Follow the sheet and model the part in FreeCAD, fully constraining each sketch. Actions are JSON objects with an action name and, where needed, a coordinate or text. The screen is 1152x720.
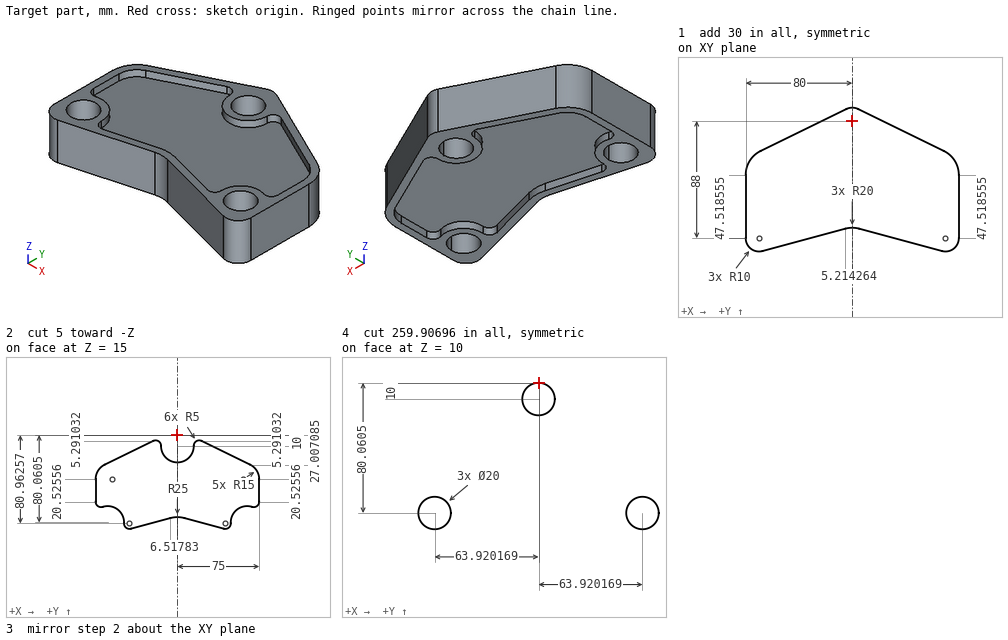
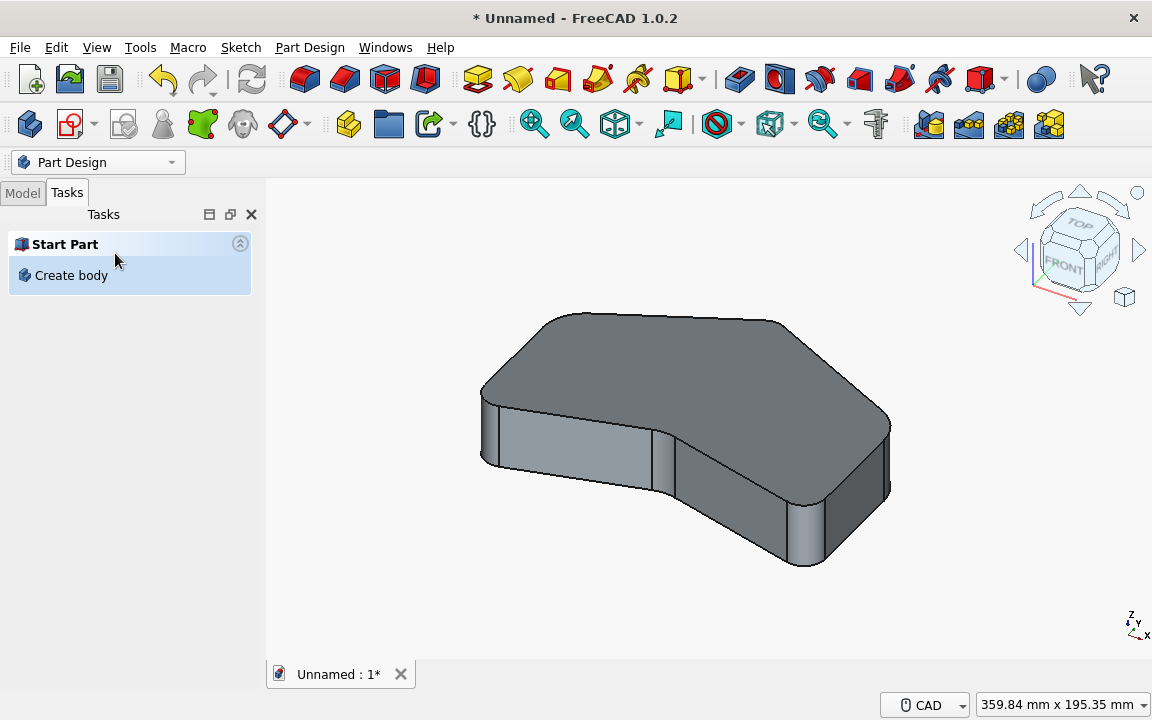
{"action": "left_click", "coordinate": [660, 371]}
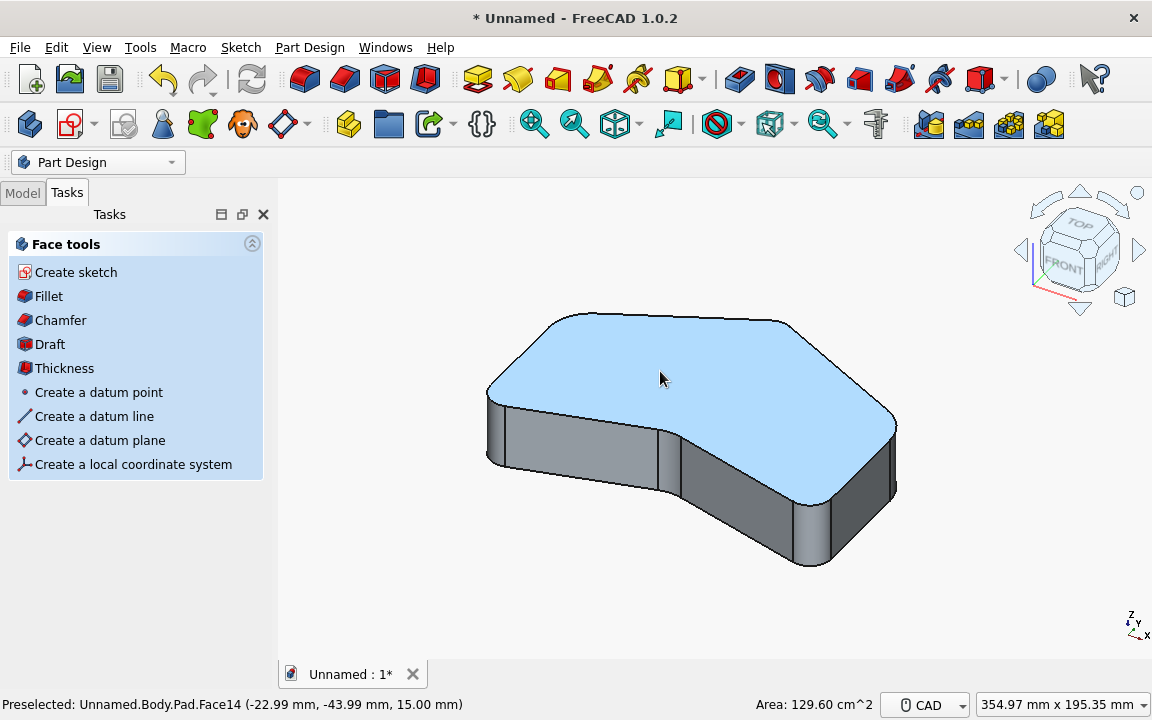
{"action": "left_click", "coordinate": [70, 124]}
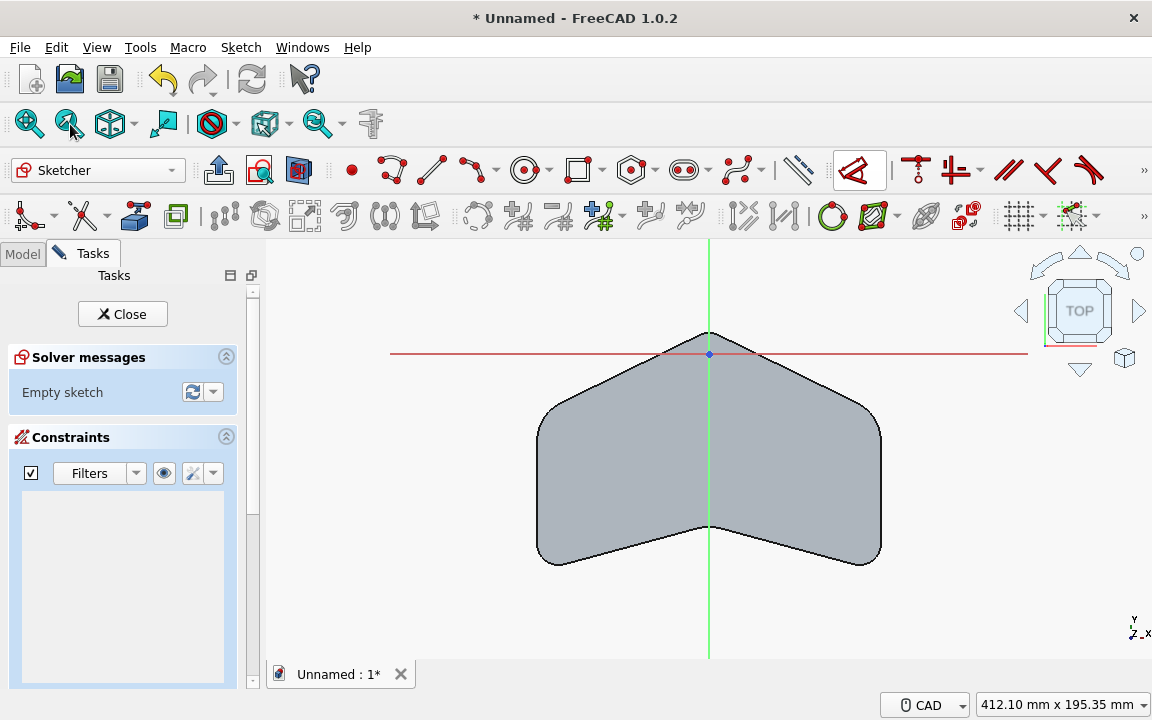
{"action": "scroll", "coordinate": [848, 442], "scroll_direction": "up", "scroll_amount": 2}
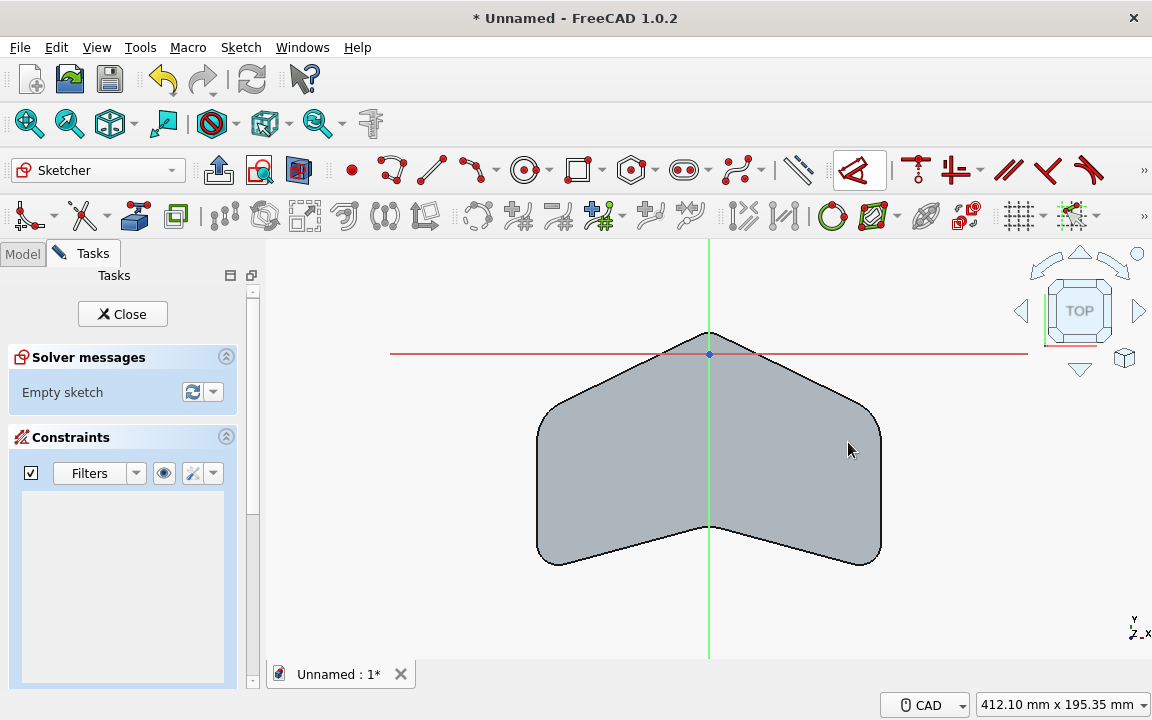
{"action": "left_click", "coordinate": [432, 170]}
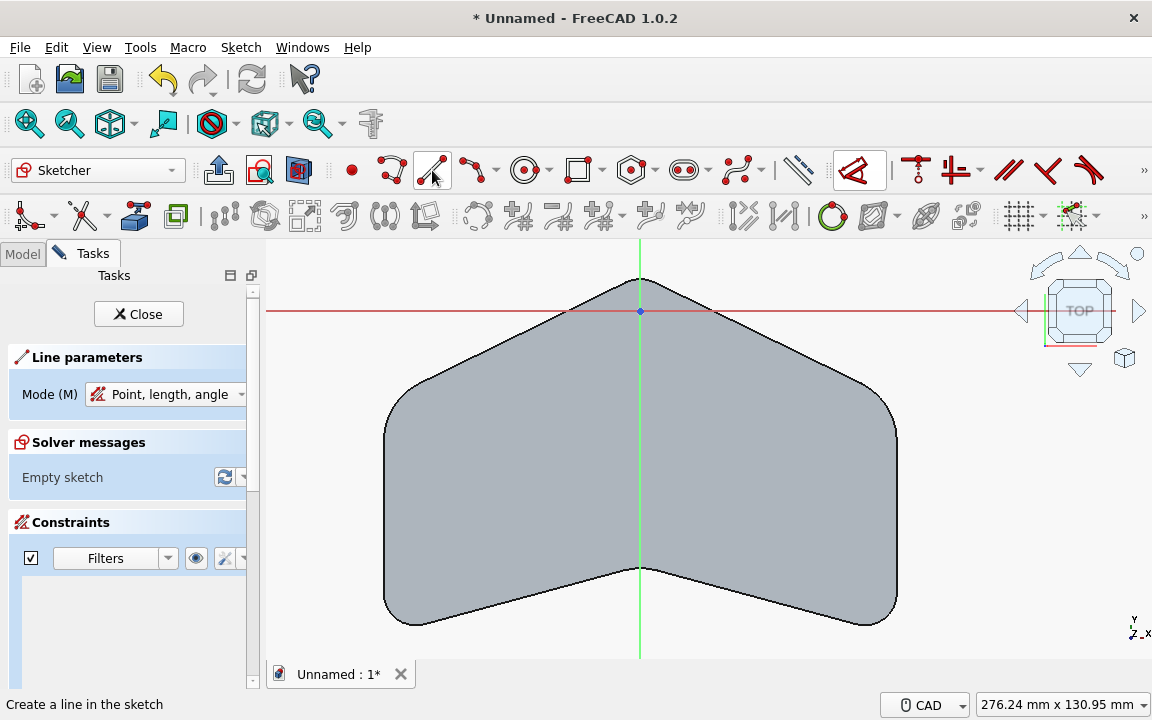
{"action": "left_click", "coordinate": [881, 507]}
{"action": "left_click", "coordinate": [881, 441]}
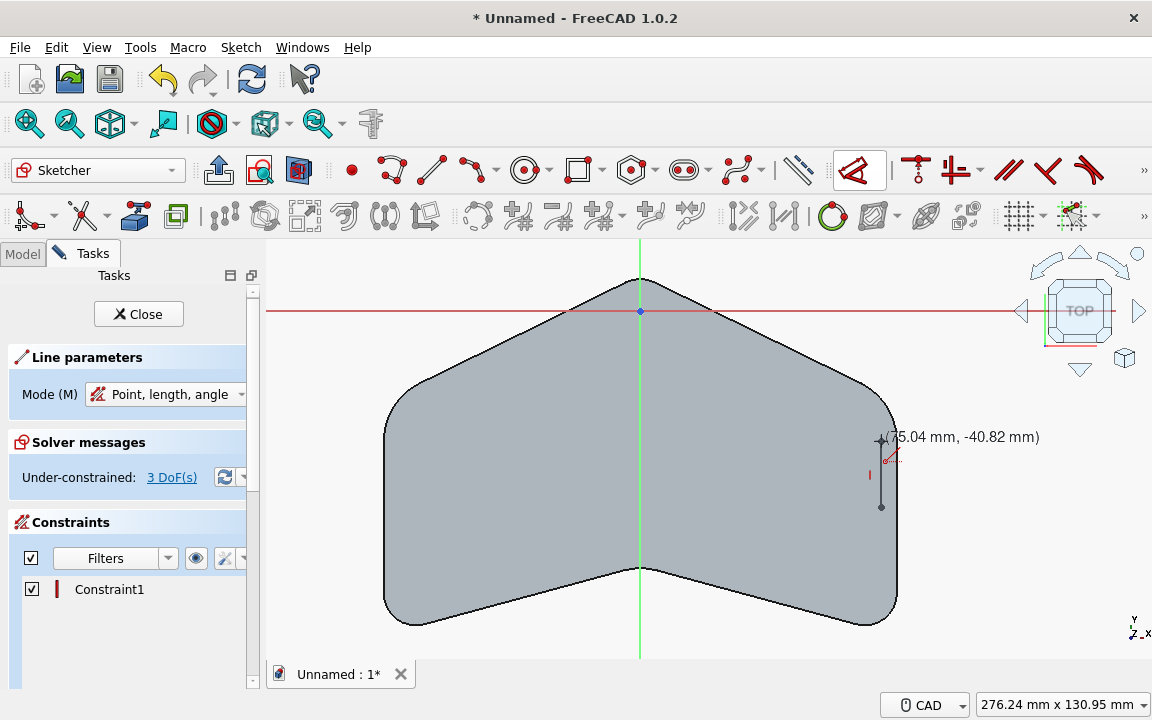
{"action": "left_click", "coordinate": [854, 398]}
{"action": "left_click", "coordinate": [712, 328]}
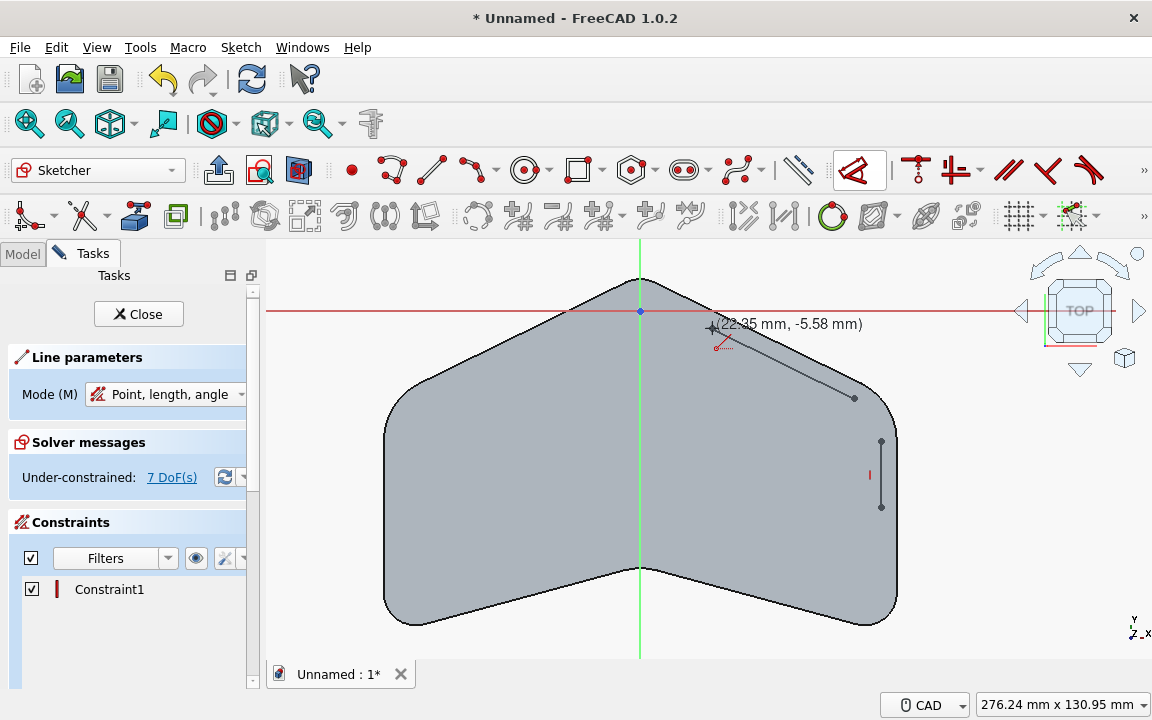
{"action": "left_click", "coordinate": [569, 328]}
{"action": "left_click", "coordinate": [427, 398]}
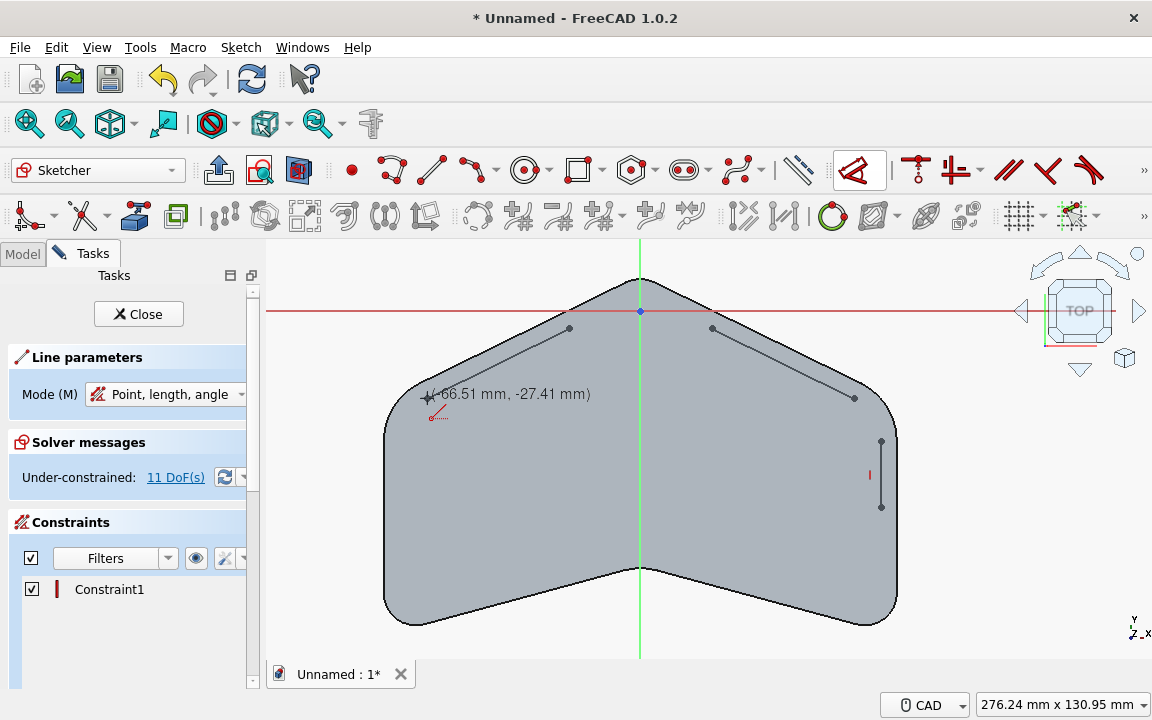
{"action": "left_click", "coordinate": [400, 441]}
{"action": "left_click", "coordinate": [400, 507]}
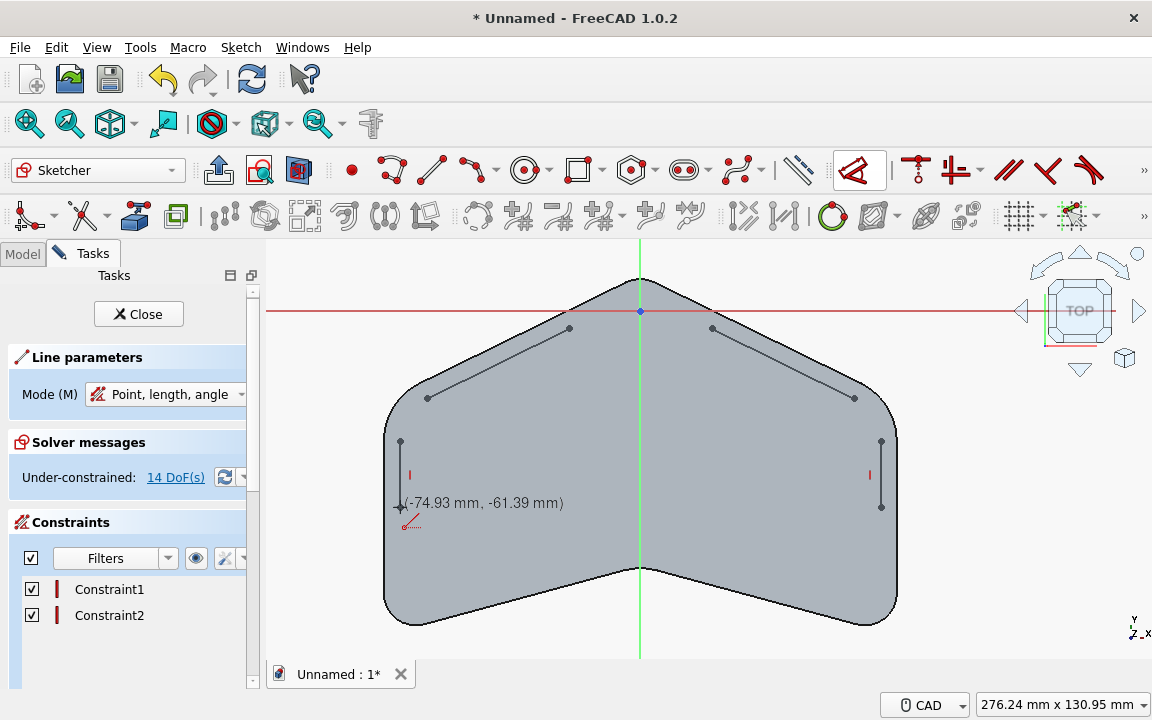
{"action": "left_click", "coordinate": [504, 586]}
{"action": "left_click", "coordinate": [619, 555]}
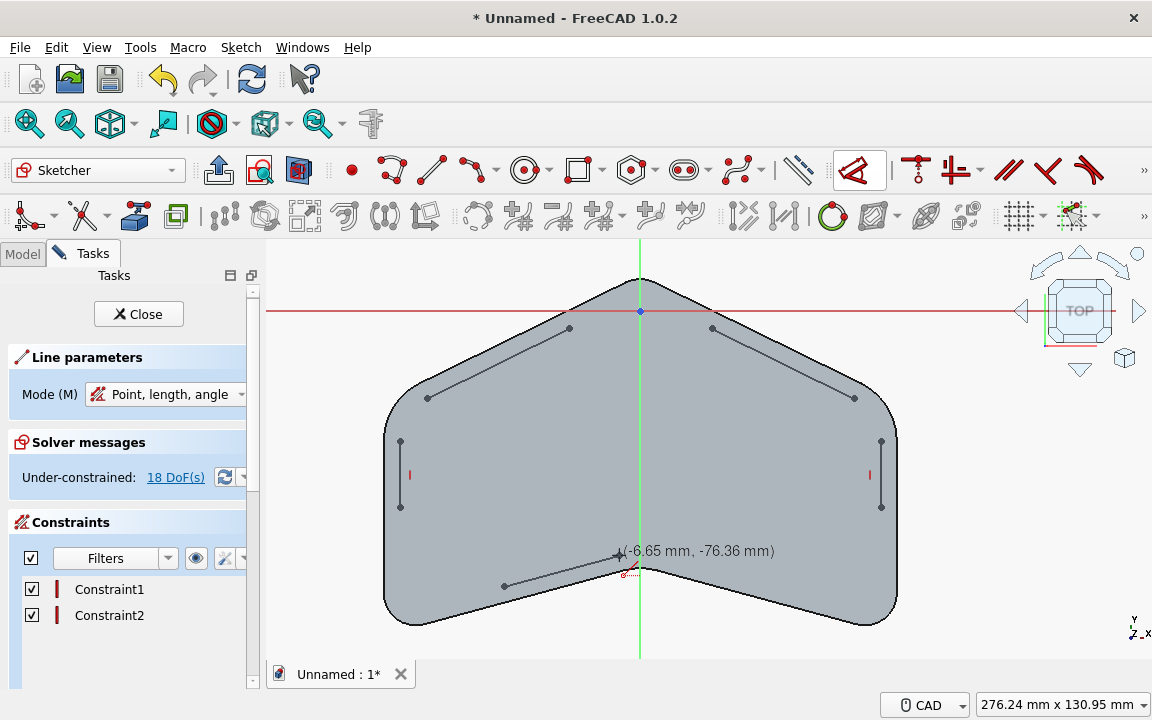
{"action": "left_click", "coordinate": [661, 555]}
{"action": "left_click", "coordinate": [777, 586]}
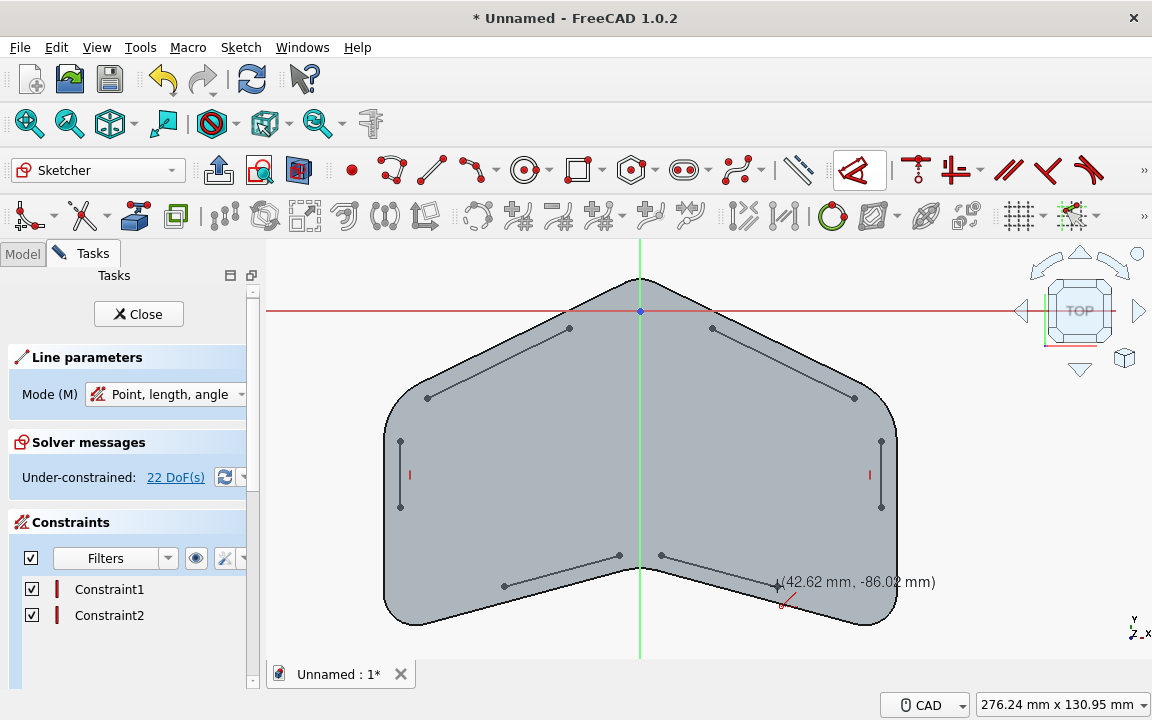
{"action": "left_click", "coordinate": [472, 170]}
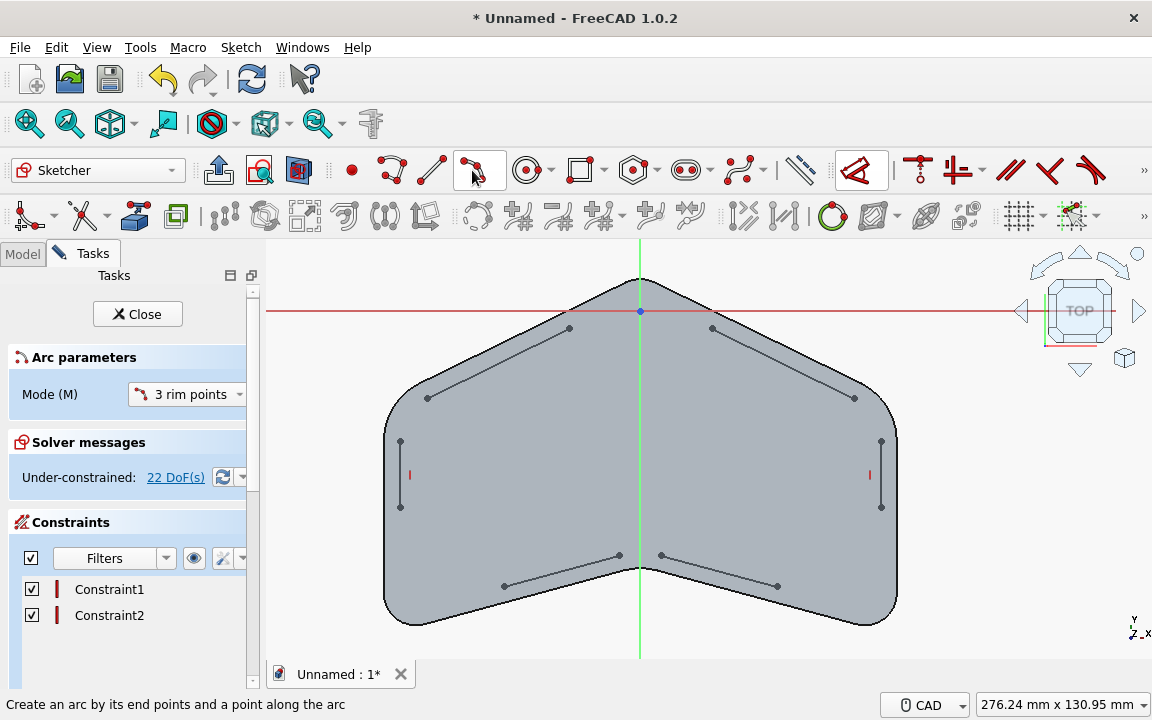
{"action": "left_click", "coordinate": [881, 442]}
{"action": "left_click", "coordinate": [854, 399]}